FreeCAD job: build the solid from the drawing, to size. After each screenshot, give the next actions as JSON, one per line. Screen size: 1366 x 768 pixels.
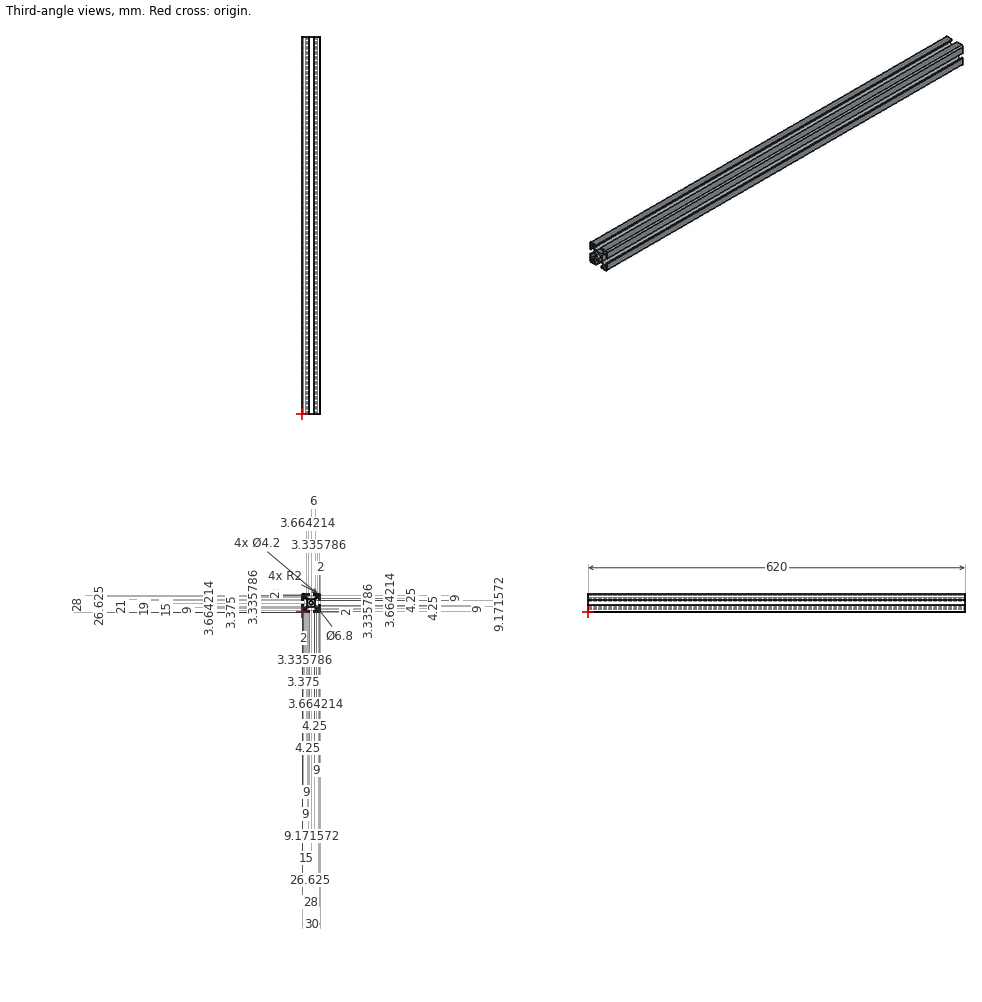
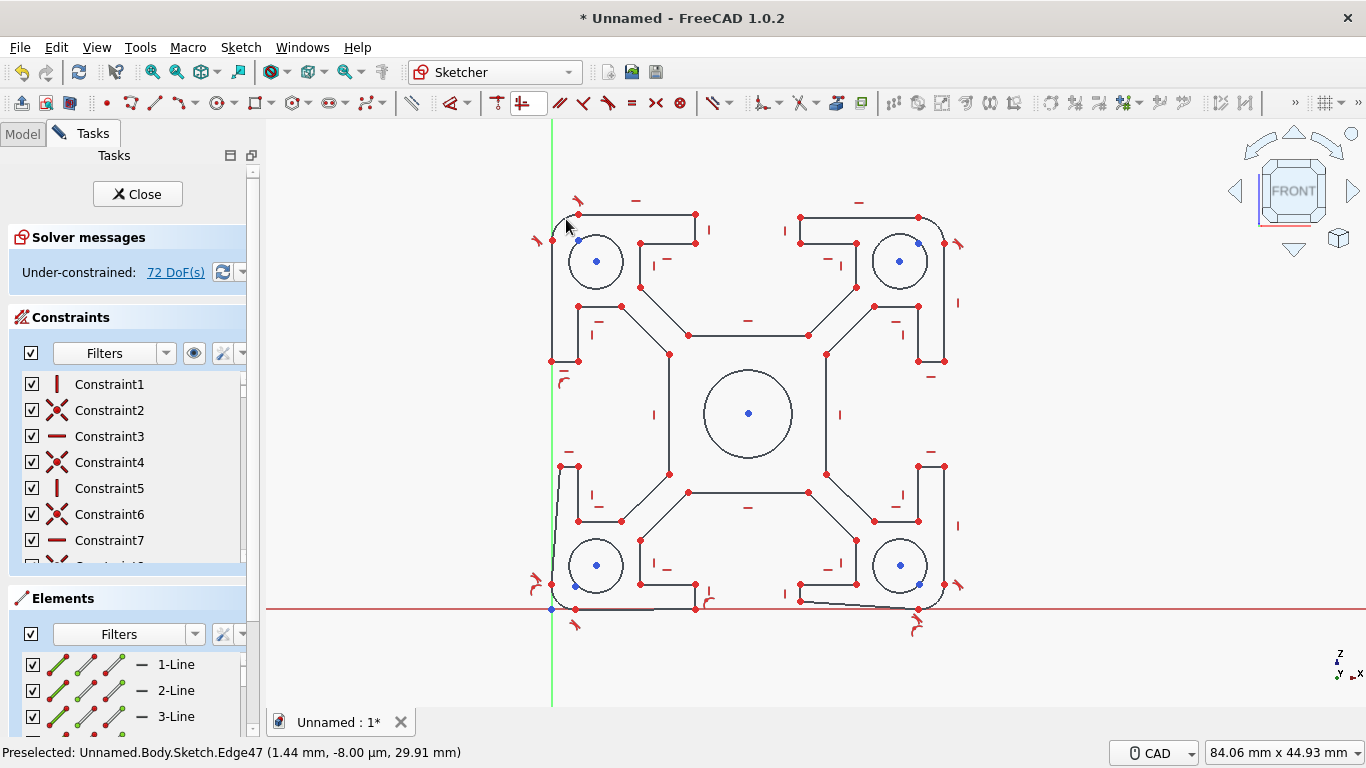
{"action": "left_click", "coordinate": [836, 218]}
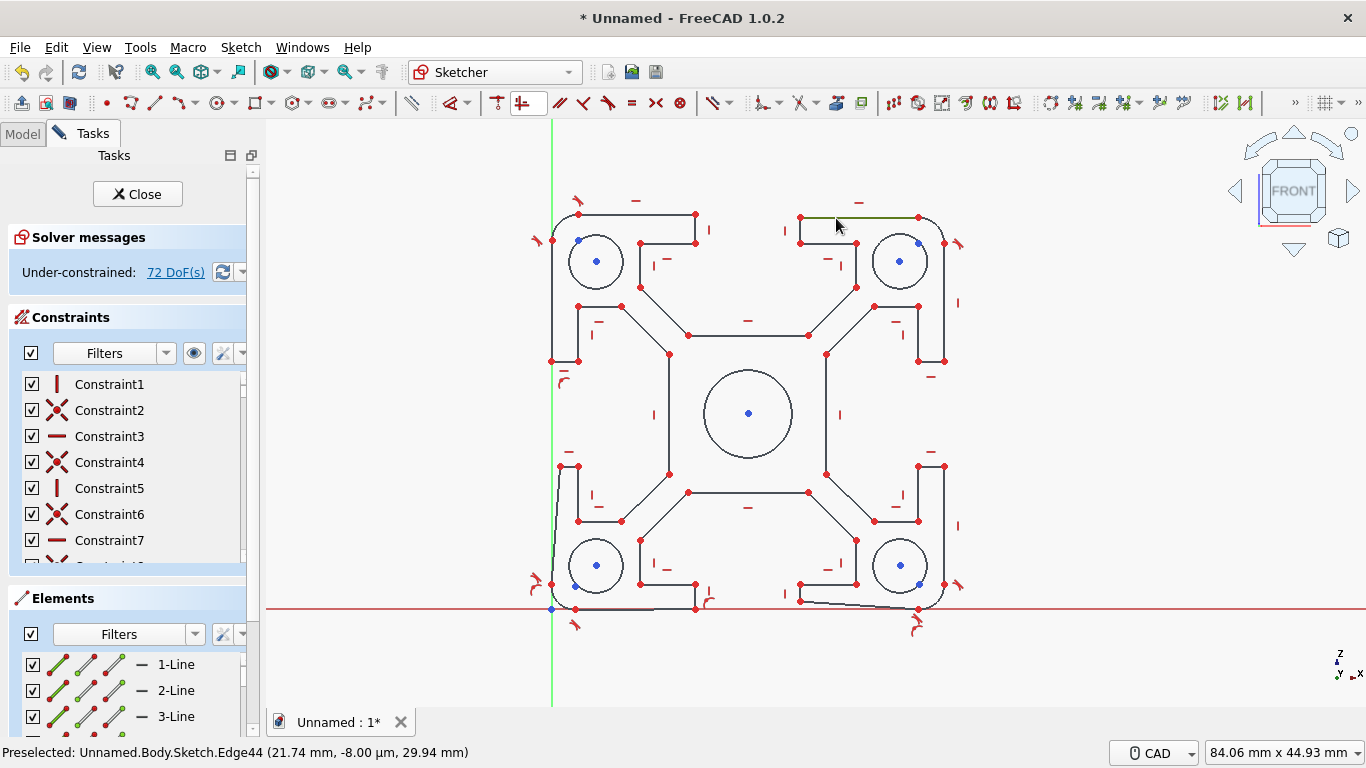
{"action": "left_click", "coordinate": [941, 232]}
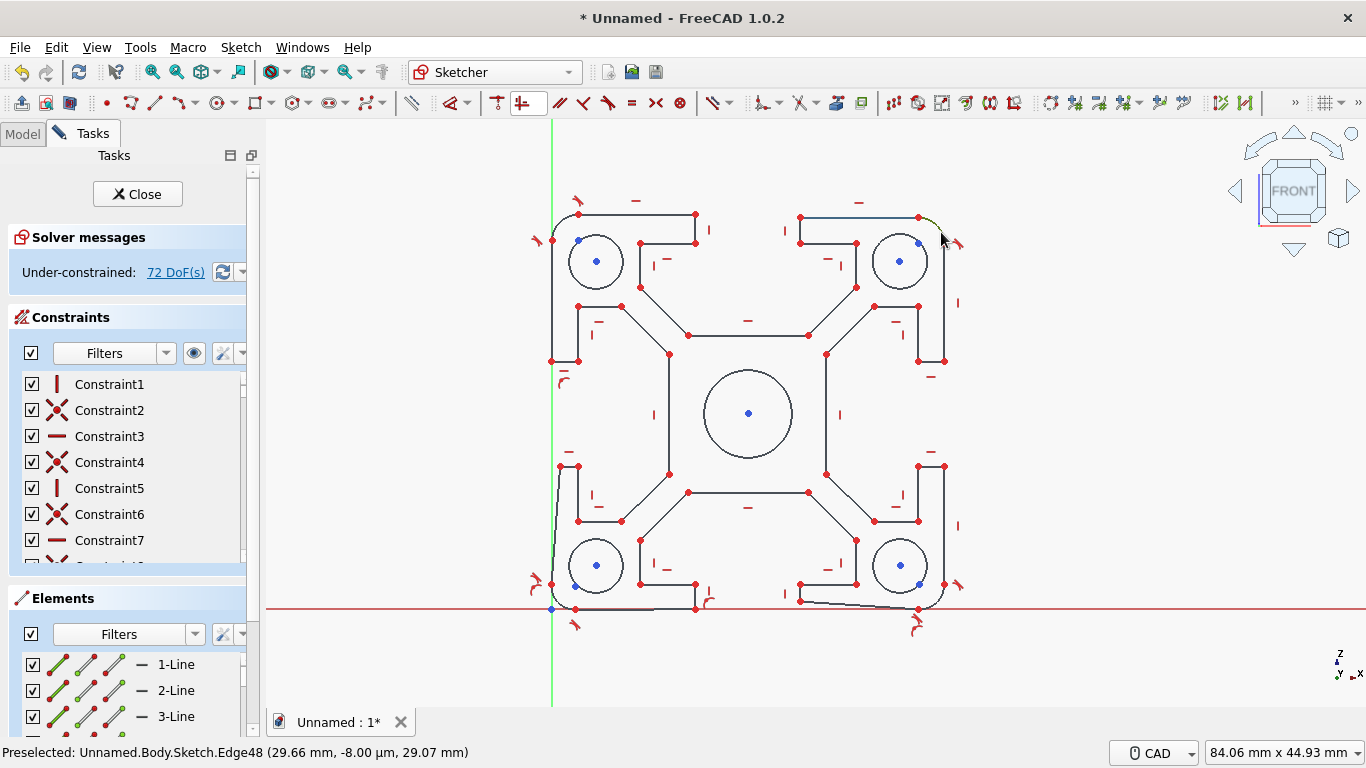
{"action": "left_click", "coordinate": [608, 104]}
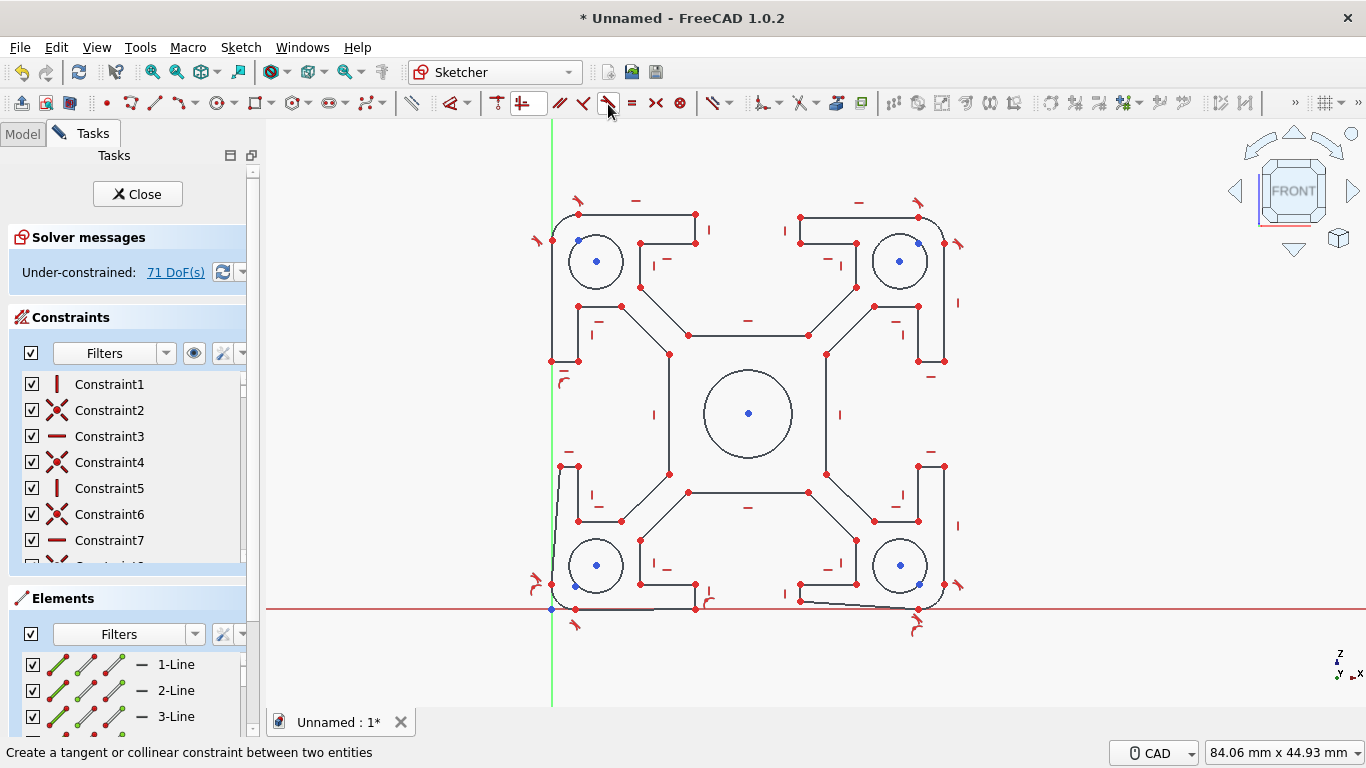
{"action": "left_click", "coordinate": [883, 607]}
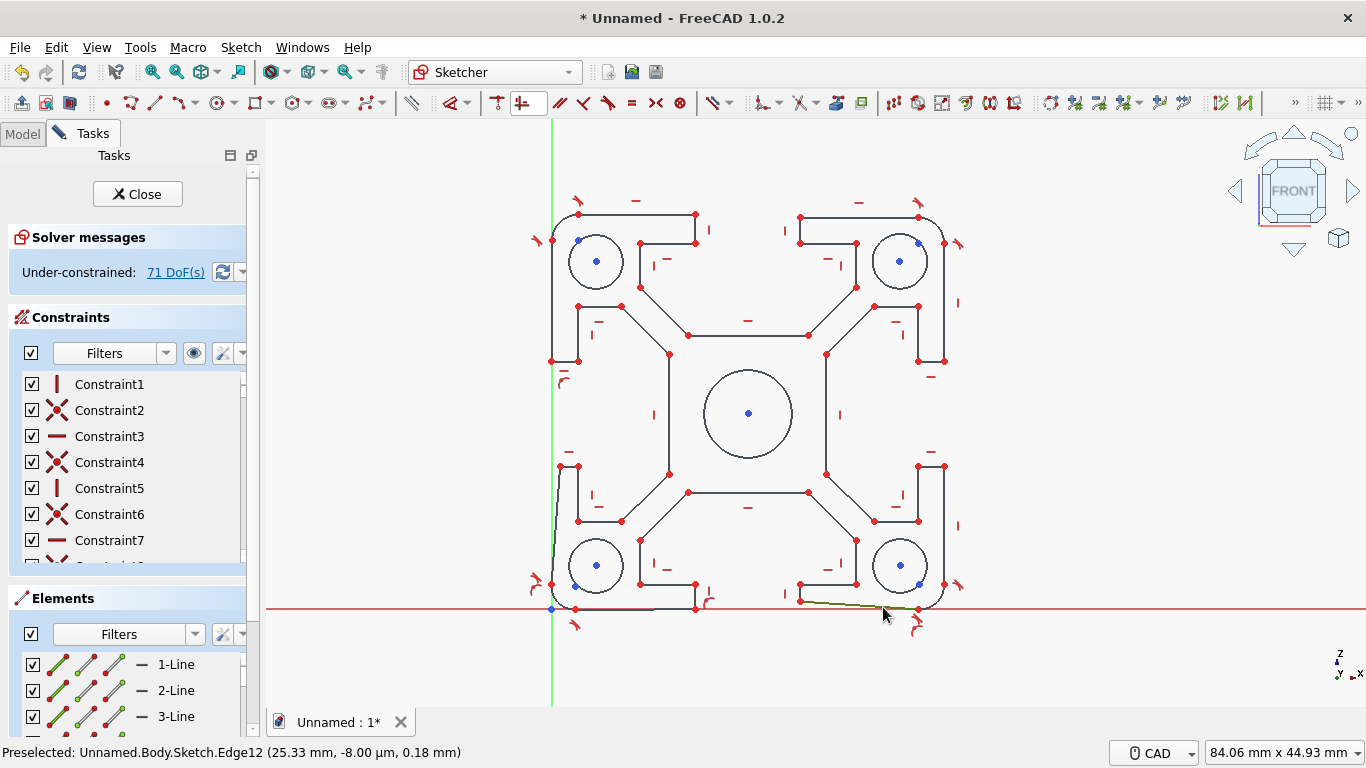
{"action": "left_click", "coordinate": [542, 104]}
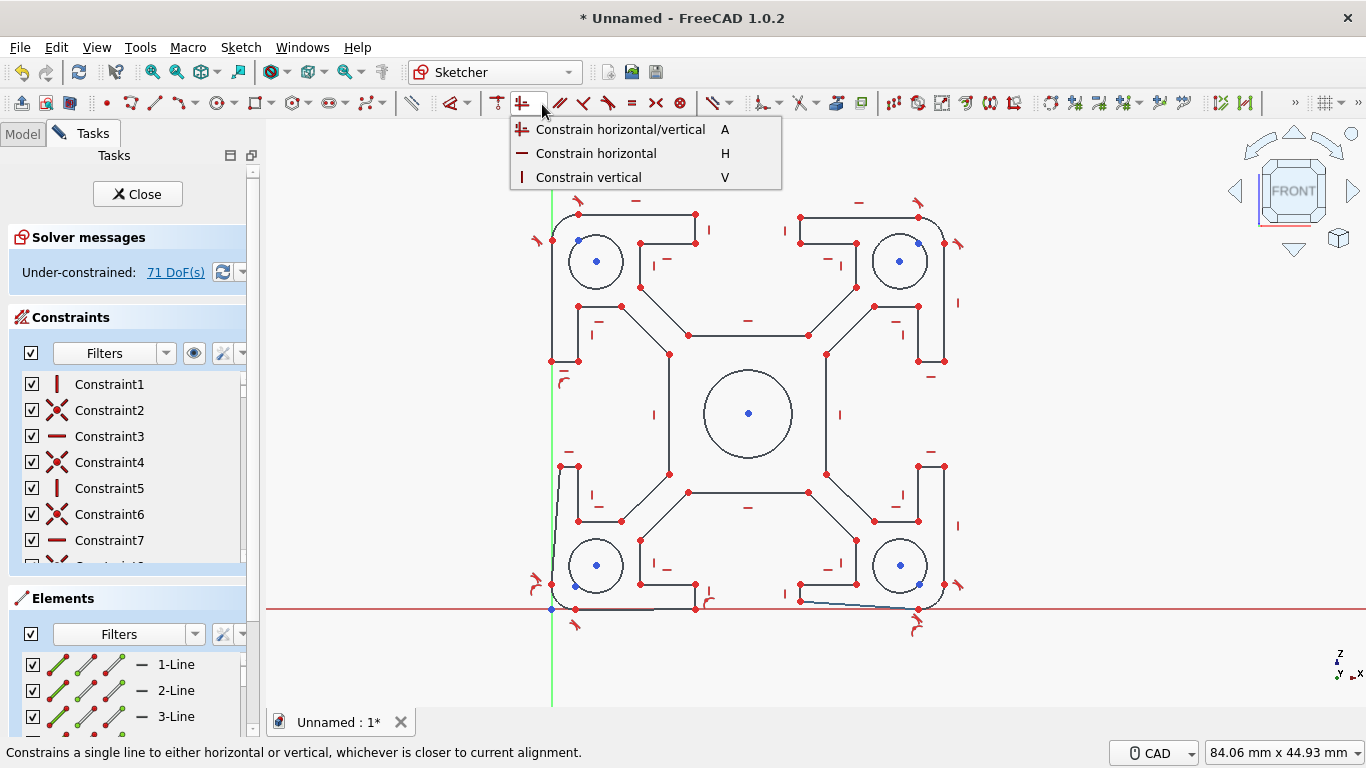
{"action": "left_click", "coordinate": [646, 153]}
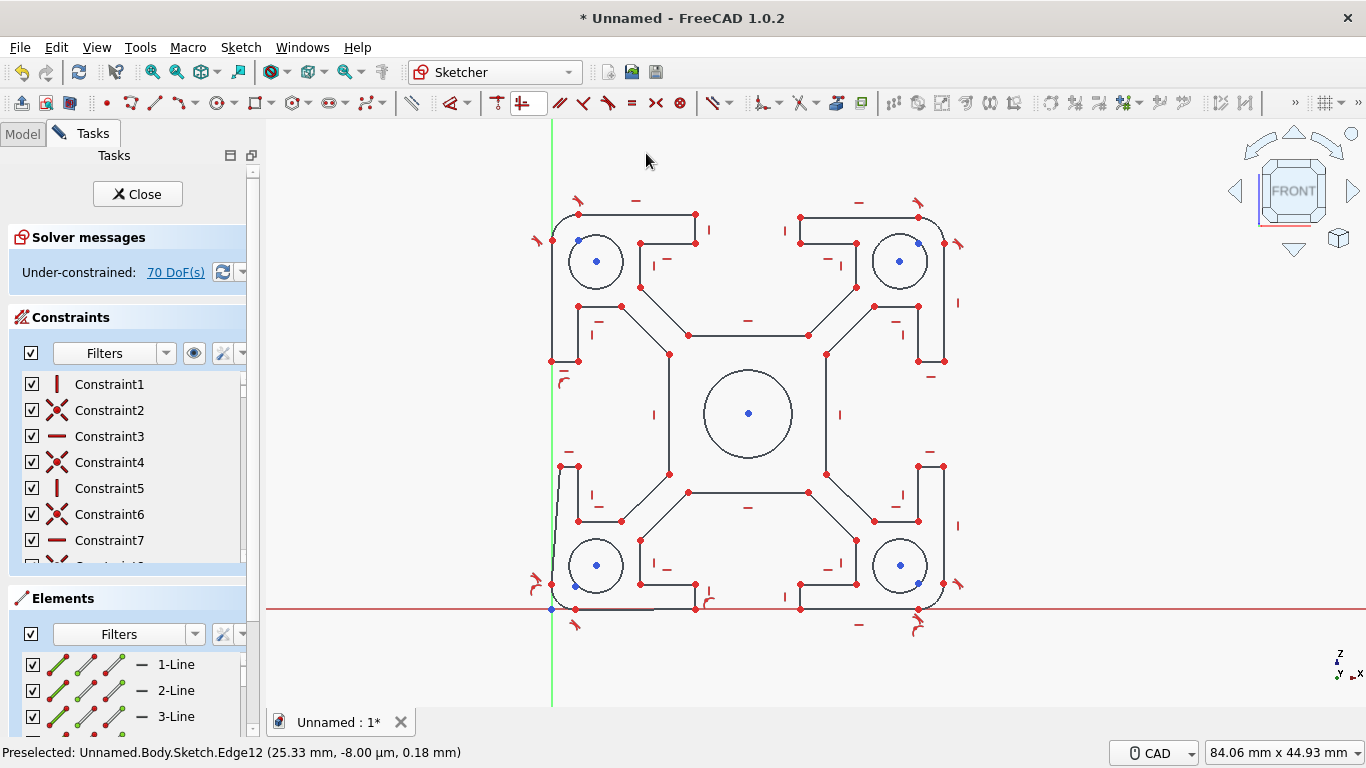
{"action": "left_click", "coordinate": [659, 609]}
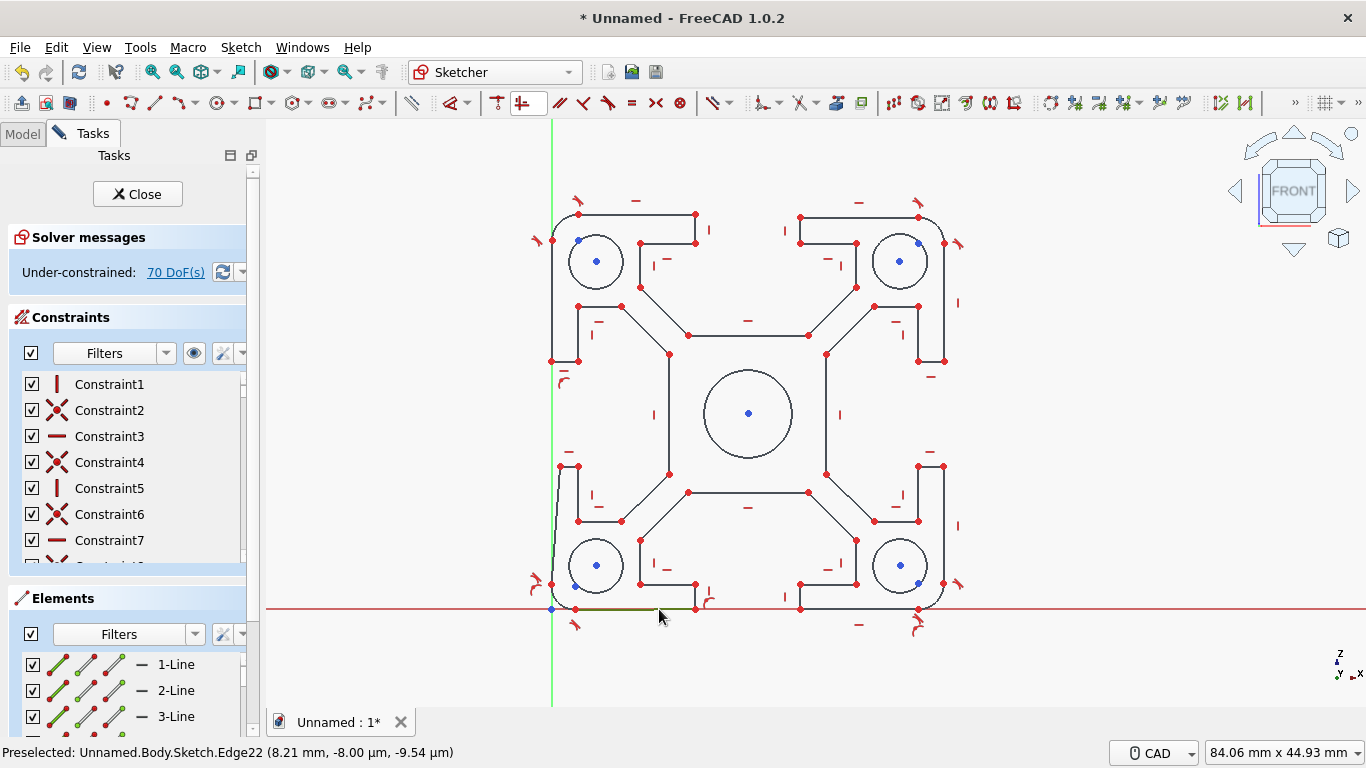
{"action": "left_click", "coordinate": [542, 104]}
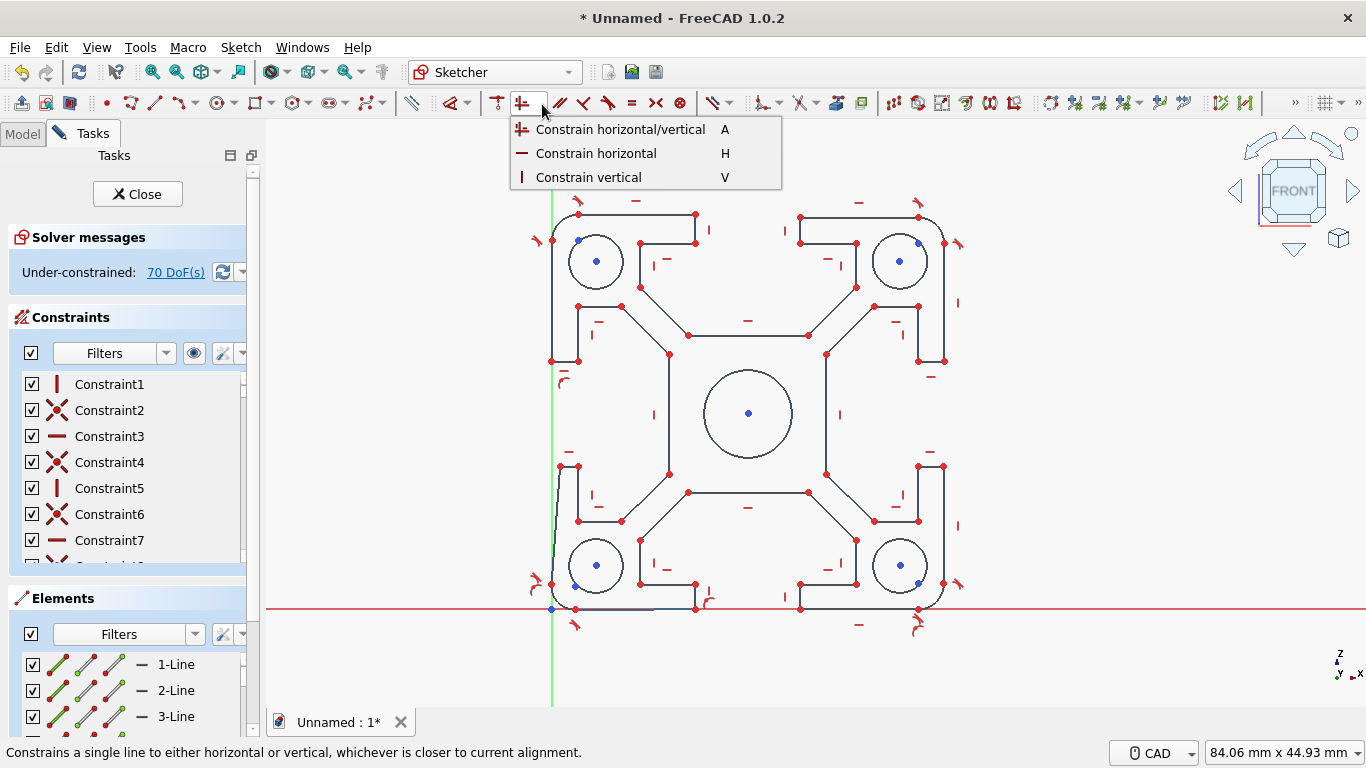
{"action": "left_click", "coordinate": [646, 153]}